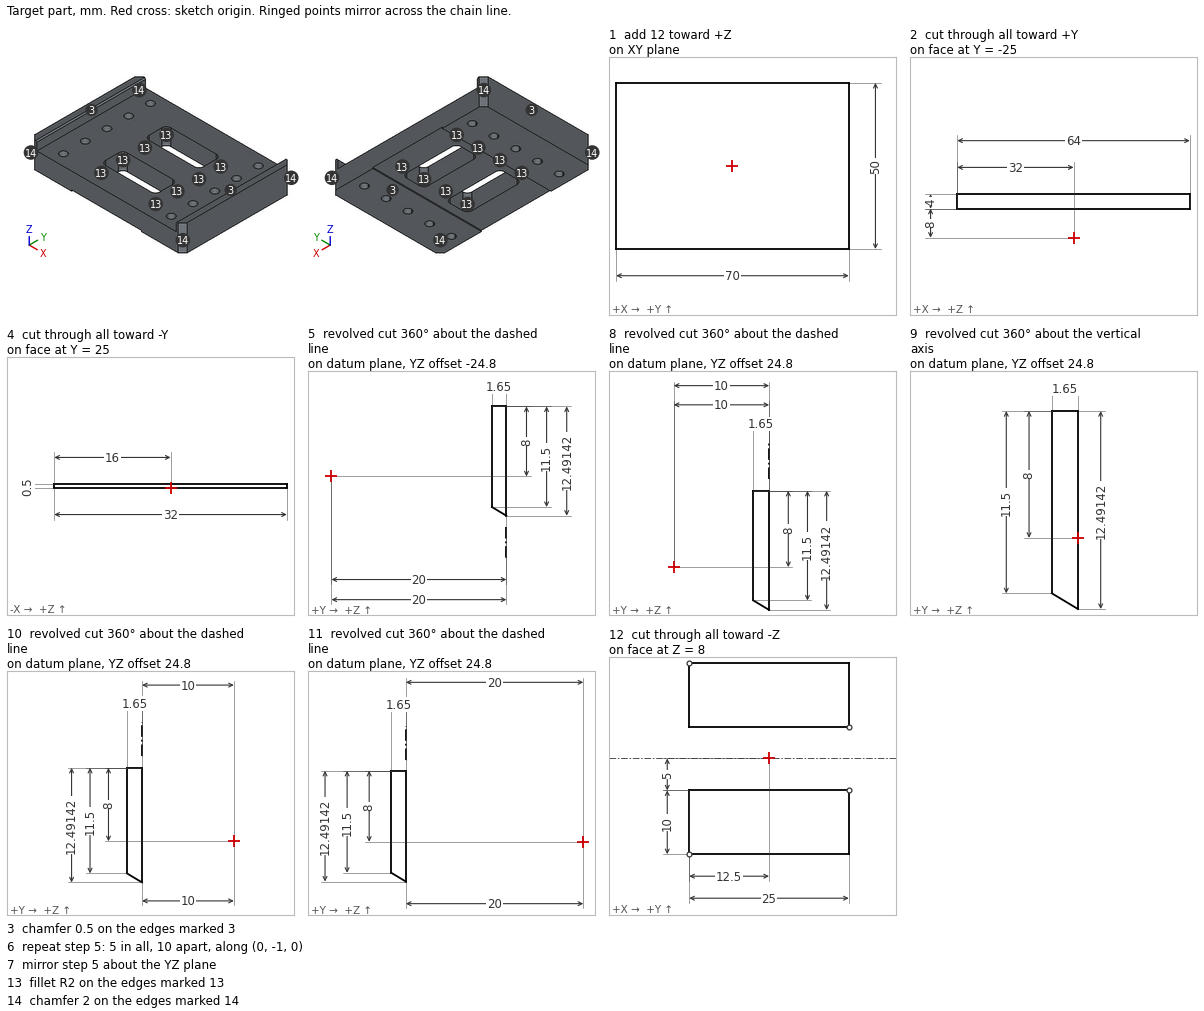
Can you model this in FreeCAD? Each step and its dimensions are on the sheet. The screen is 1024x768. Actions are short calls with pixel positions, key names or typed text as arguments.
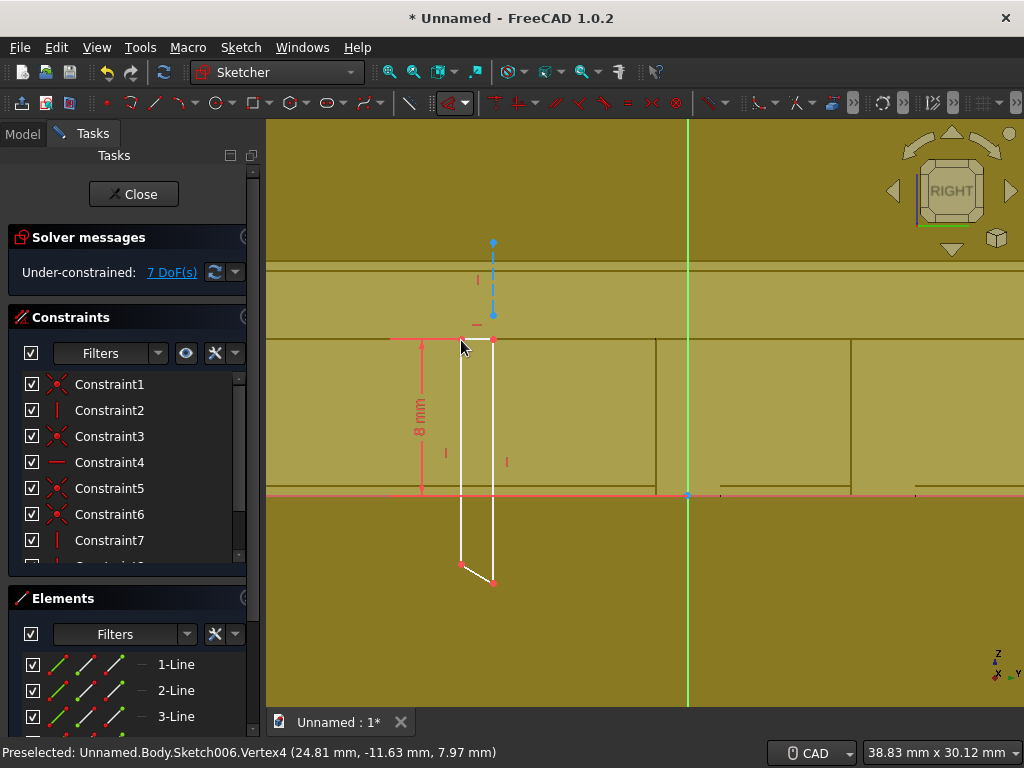
click(493, 584)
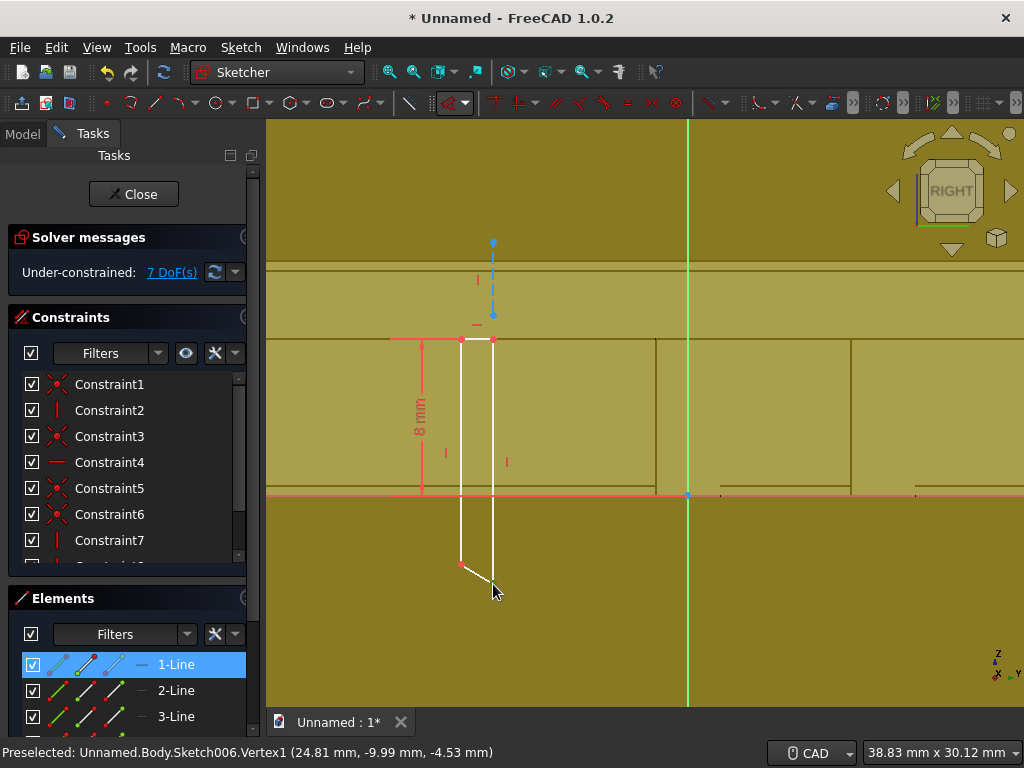
key(l)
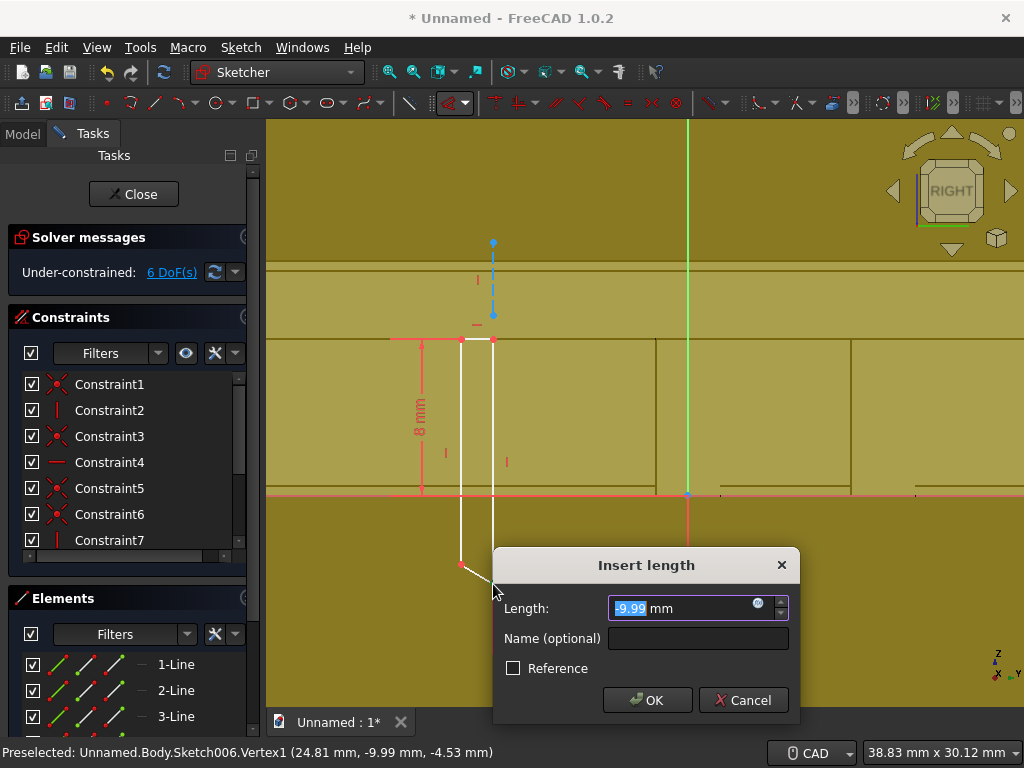
text(-10)
key(Return)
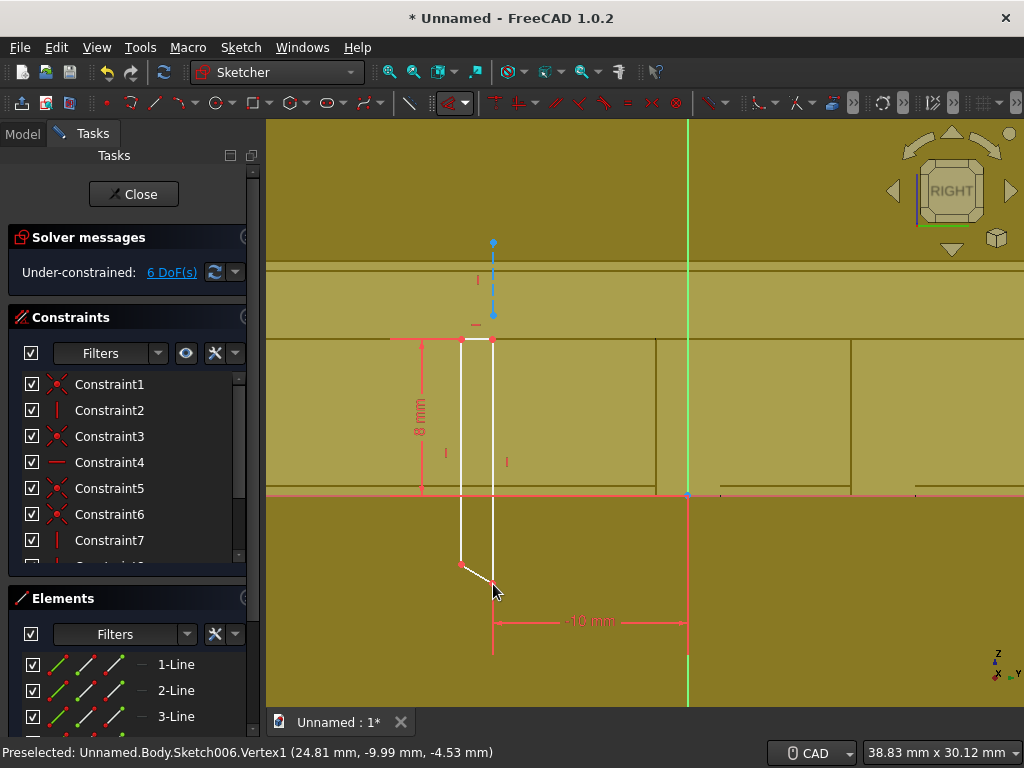
click(493, 316)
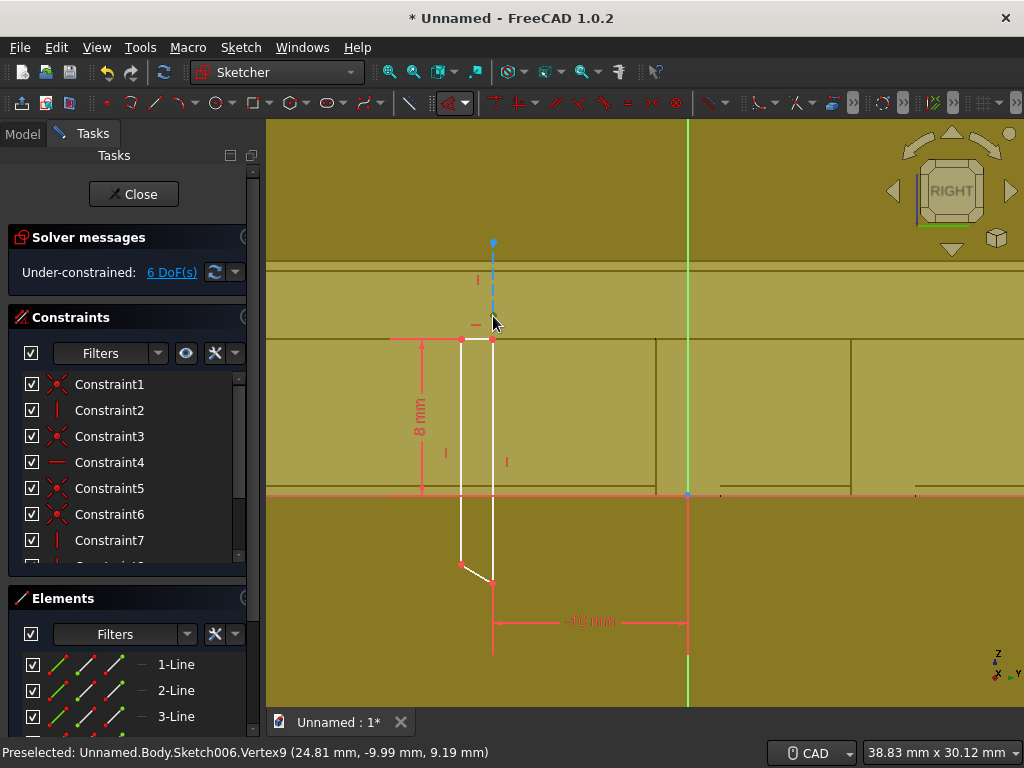
key(l)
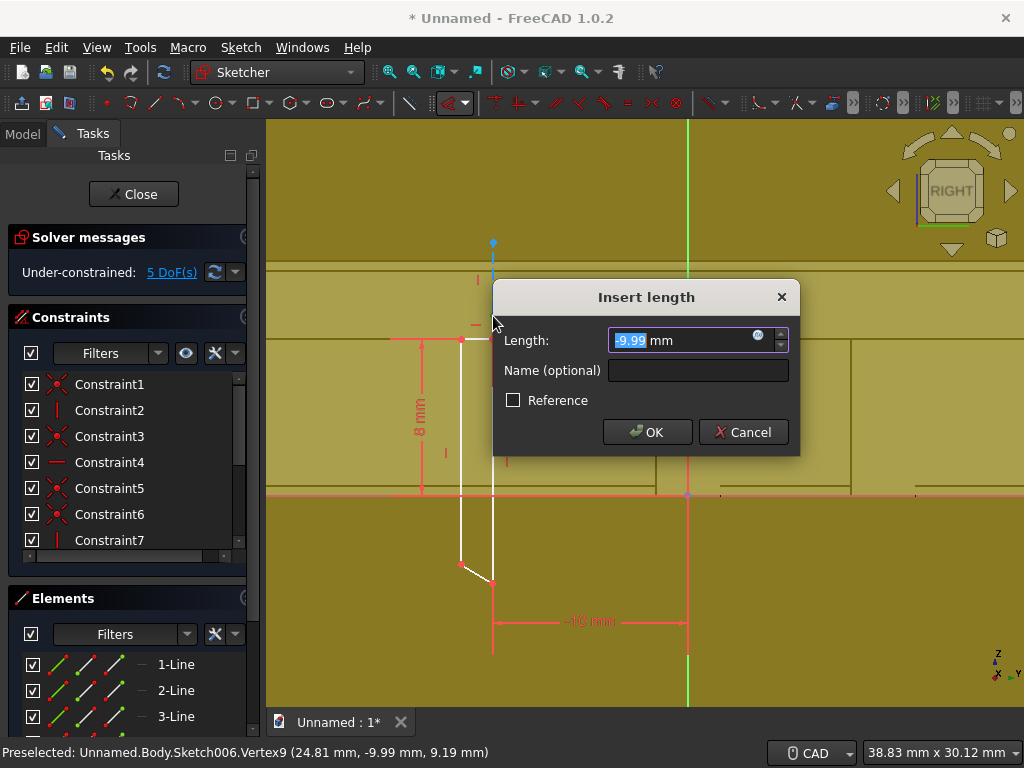
text(-10)
key(Return)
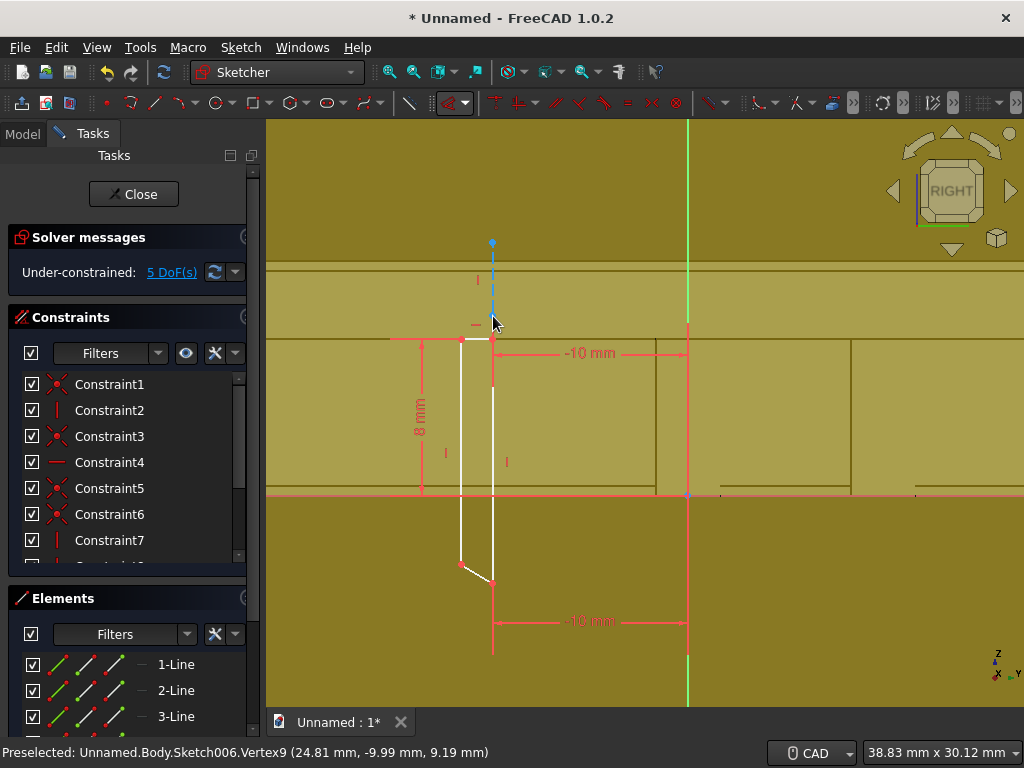
click(461, 497)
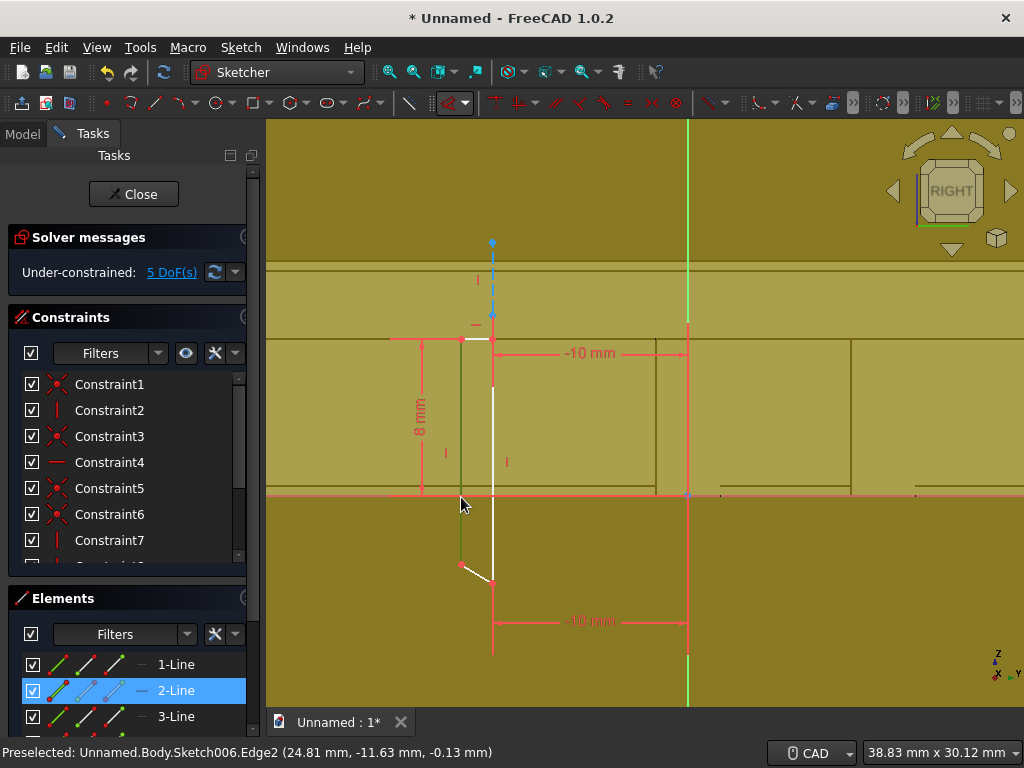
key(i)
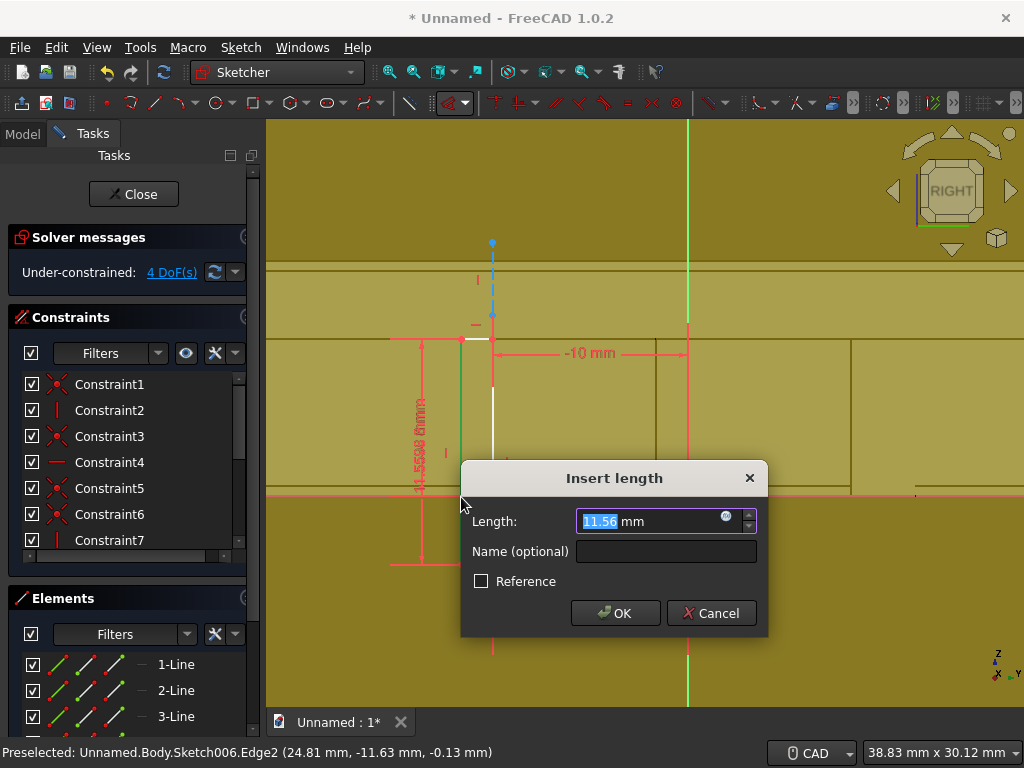
text(11.5)
key(Return)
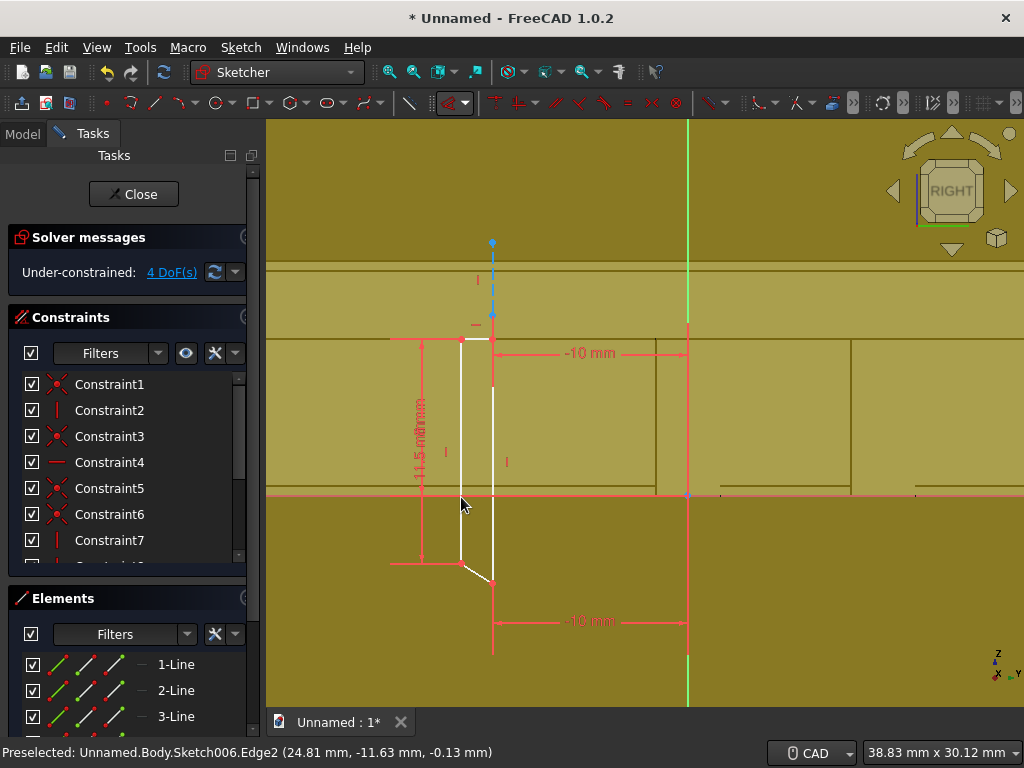
scroll(471, 339, up, 2)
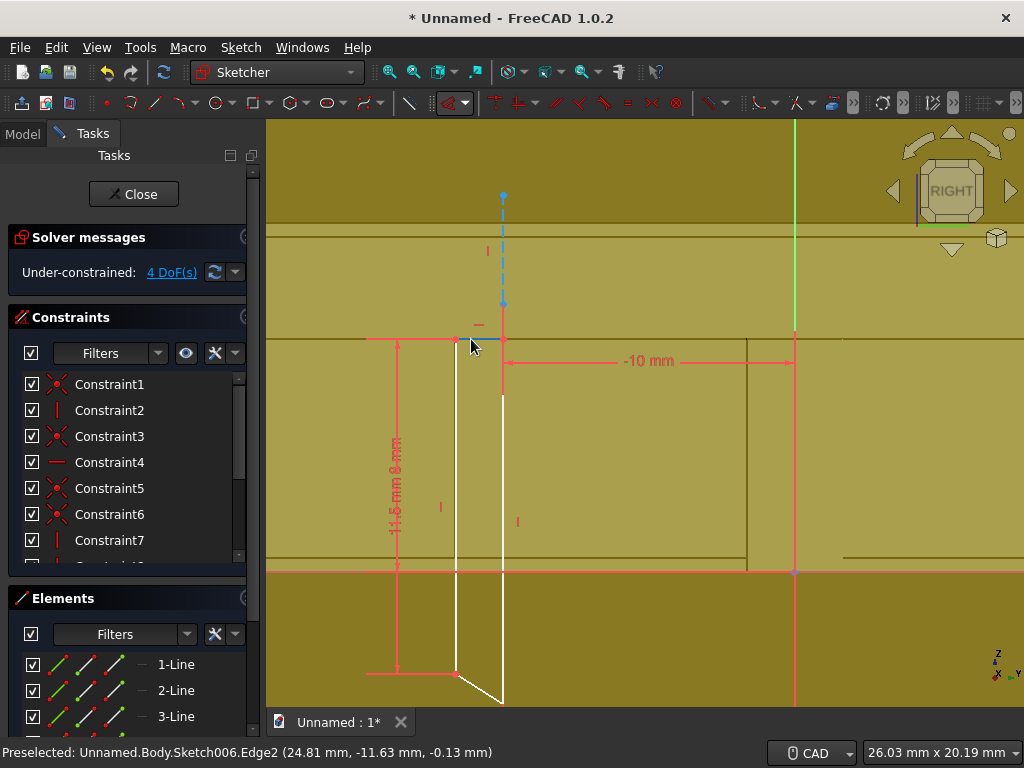
click(470, 339)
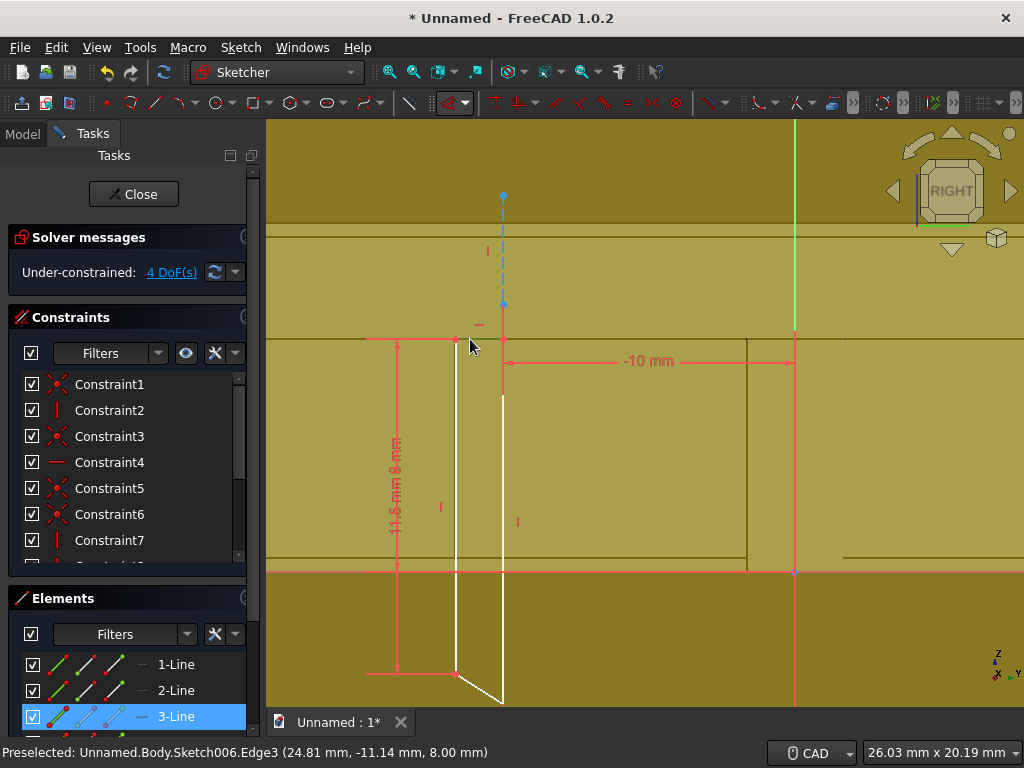
key(l)